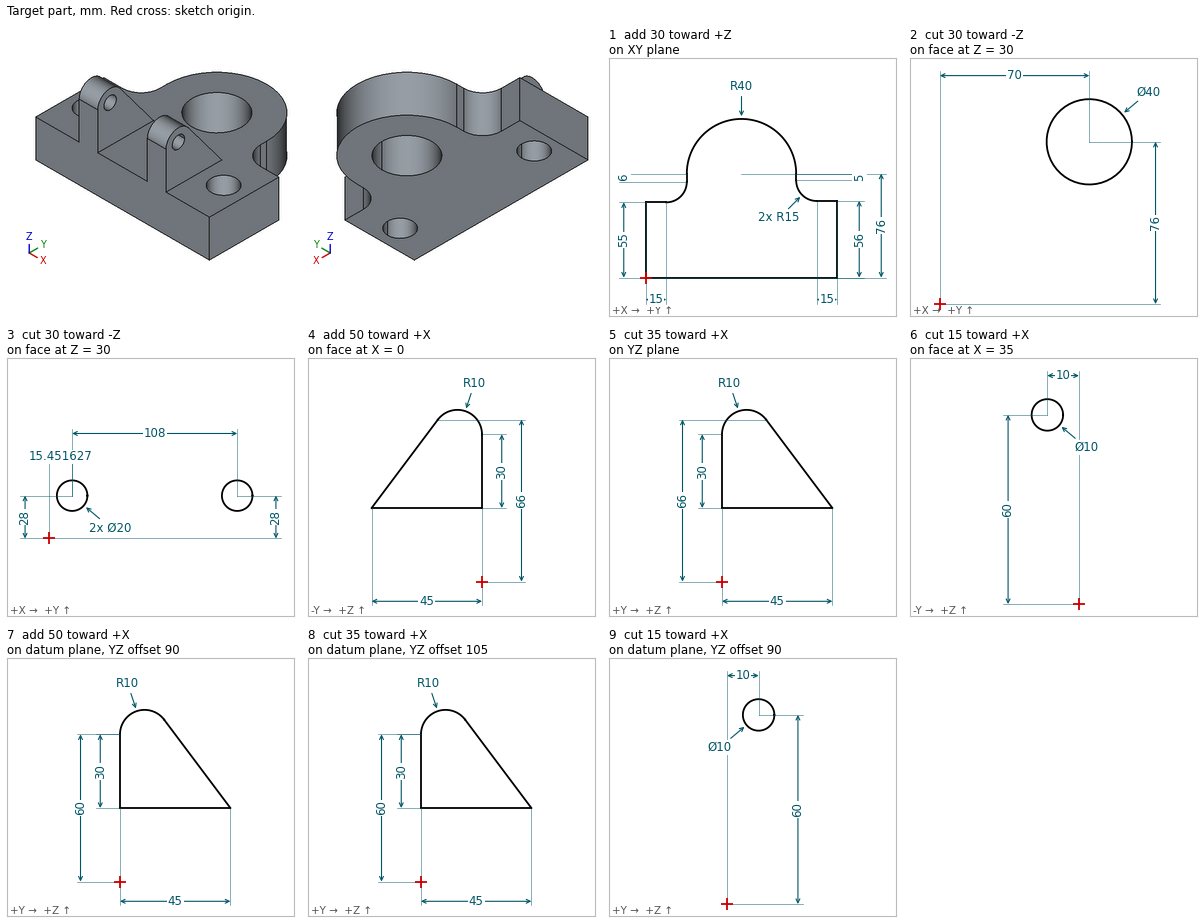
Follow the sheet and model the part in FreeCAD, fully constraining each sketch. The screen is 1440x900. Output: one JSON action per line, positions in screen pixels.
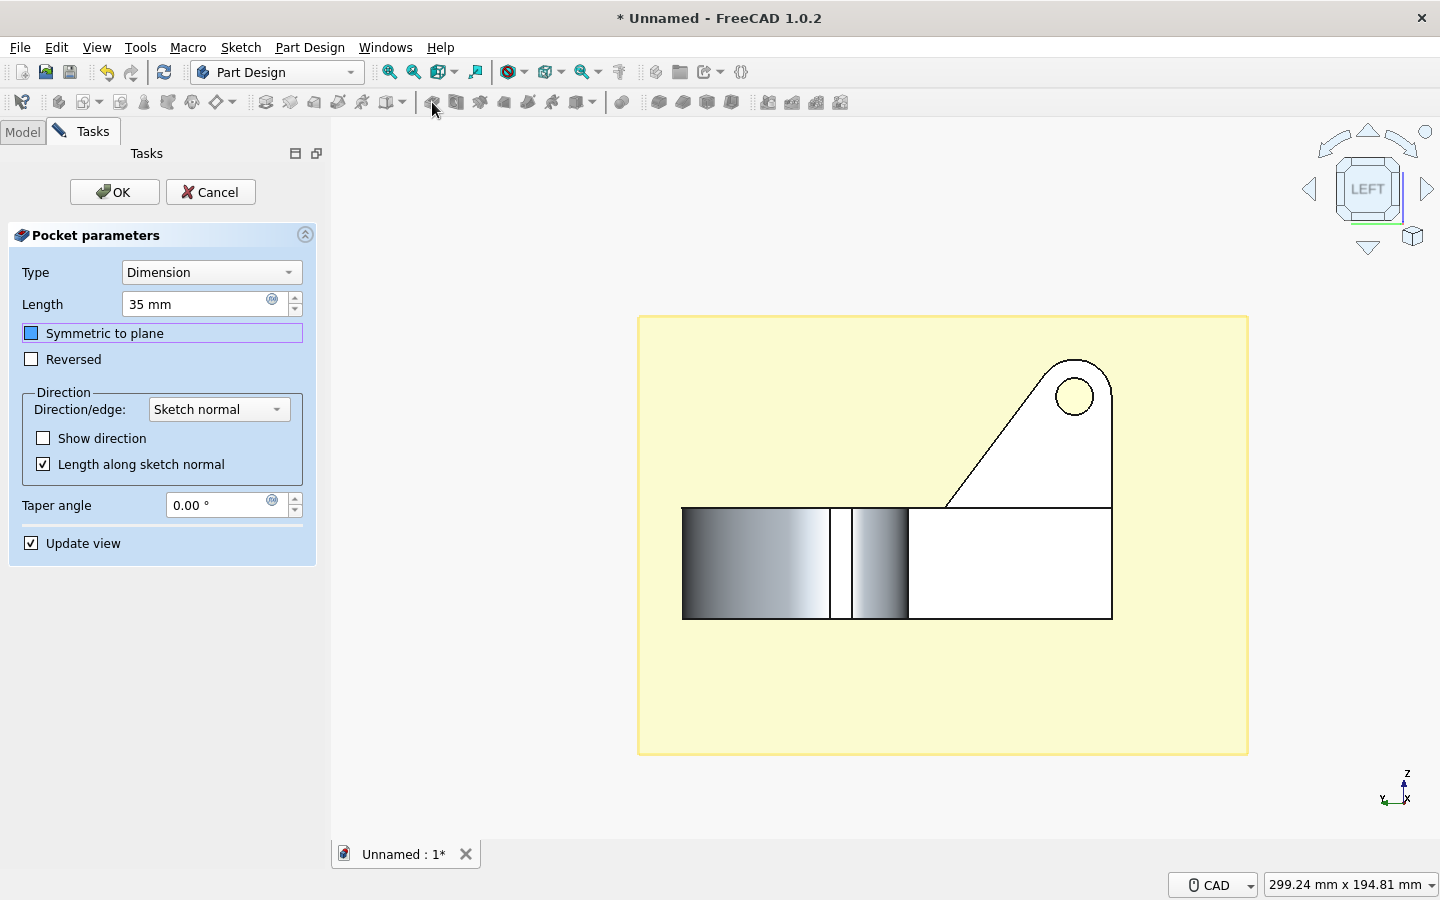
{"action": "left_click", "coordinate": [30, 359]}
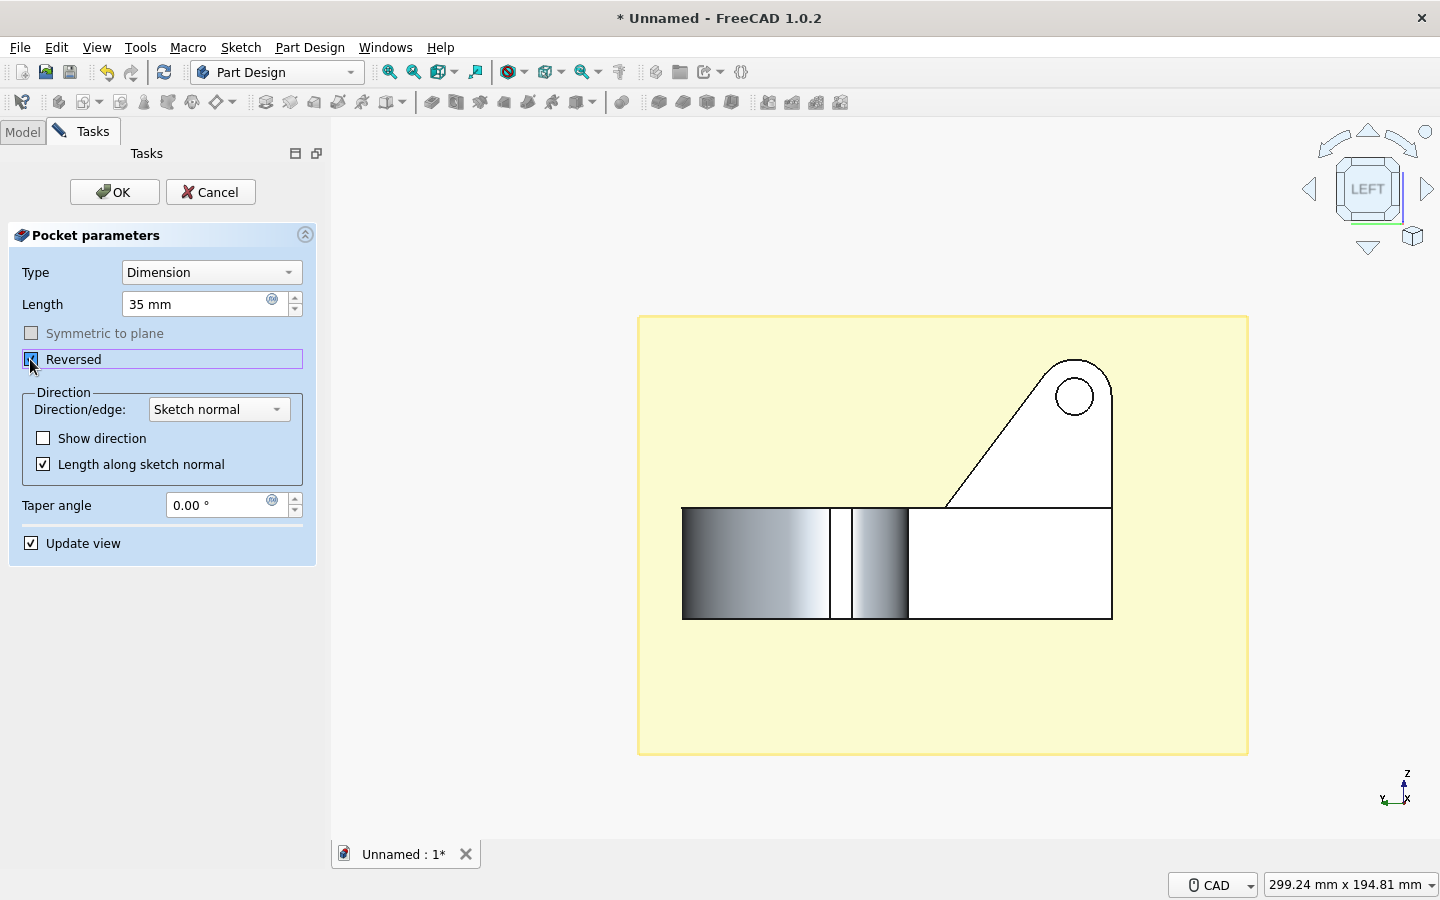
{"action": "left_click", "coordinate": [115, 192]}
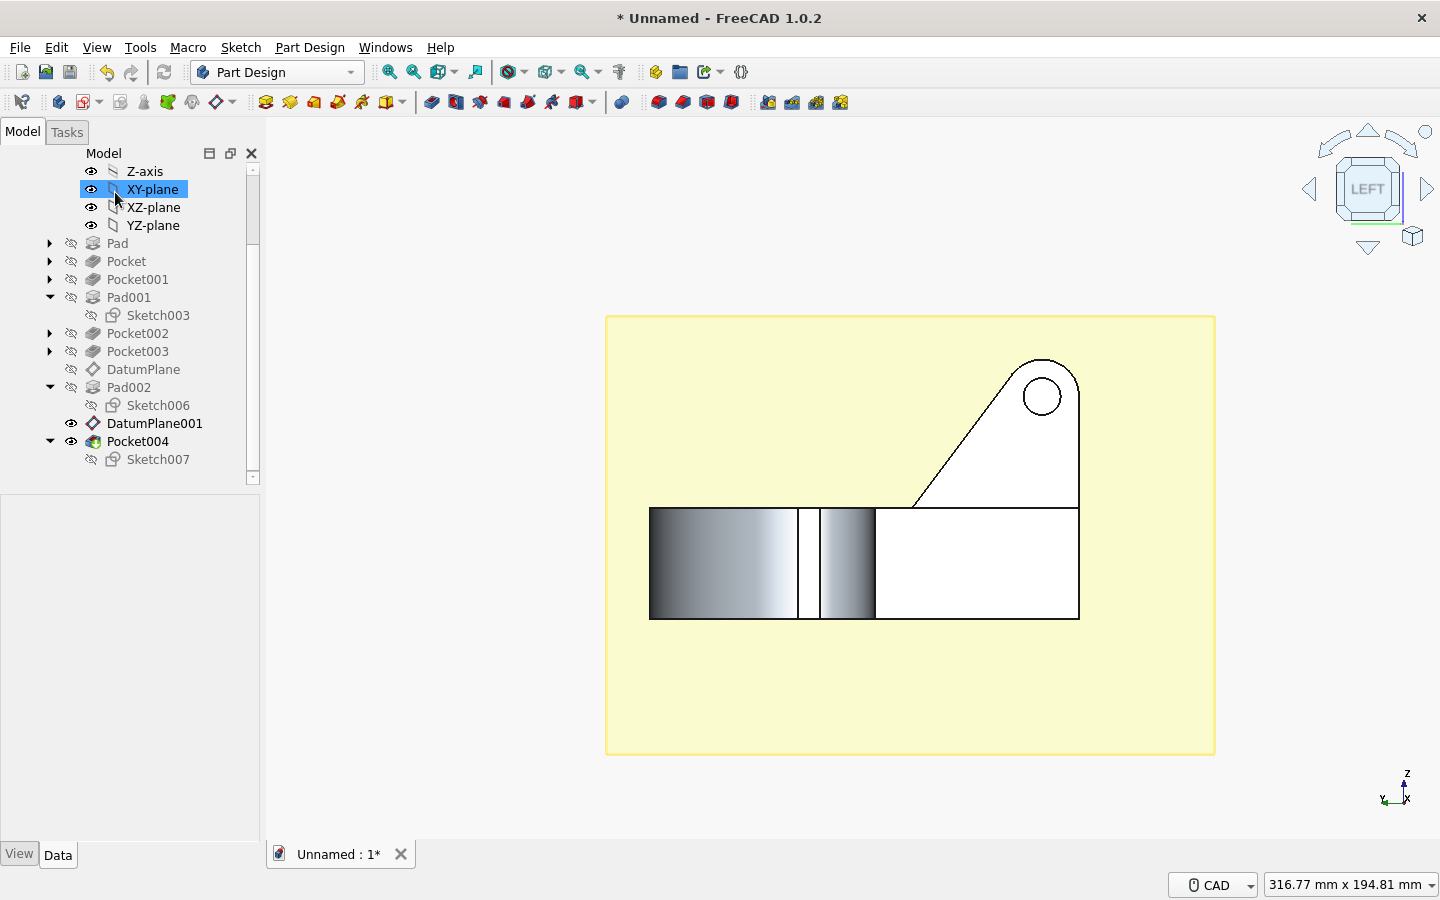
{"action": "left_click", "coordinate": [116, 423]}
{"action": "key", "text": "space"}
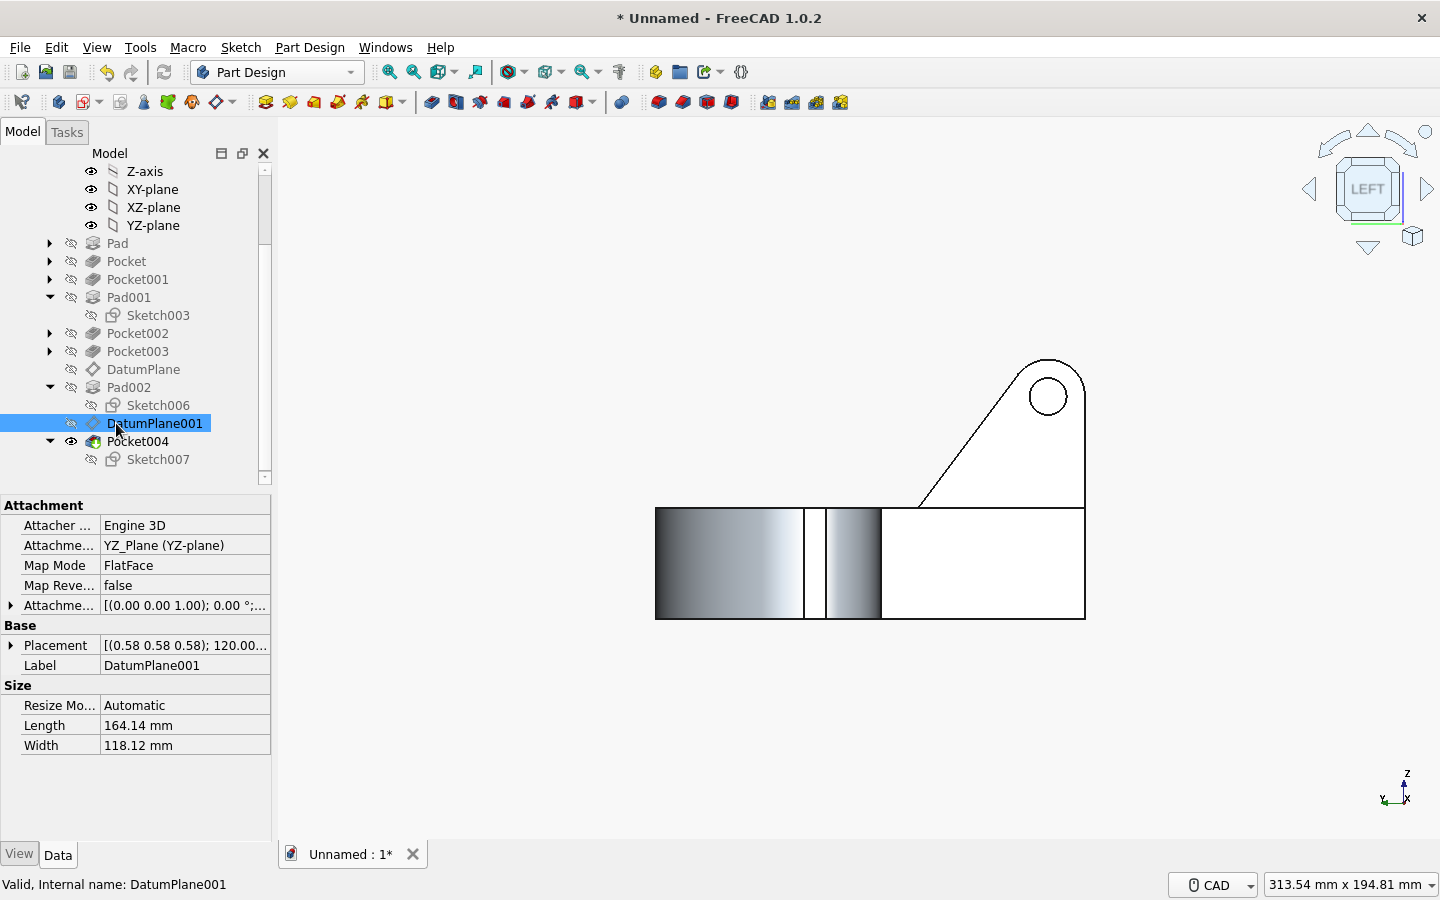
{"action": "key", "text": "v f"}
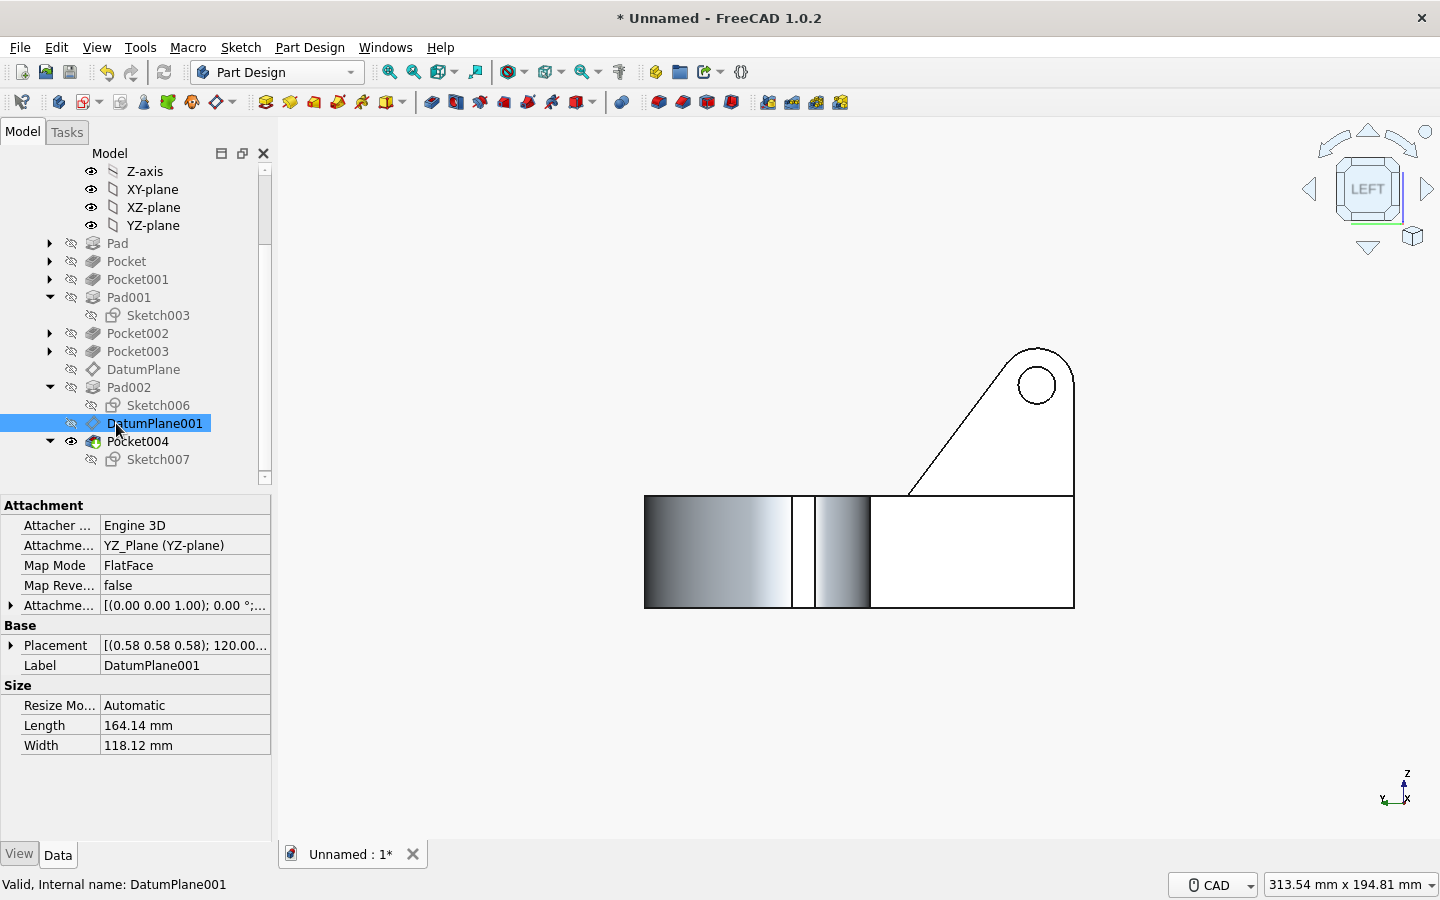
{"action": "key", "text": "2"}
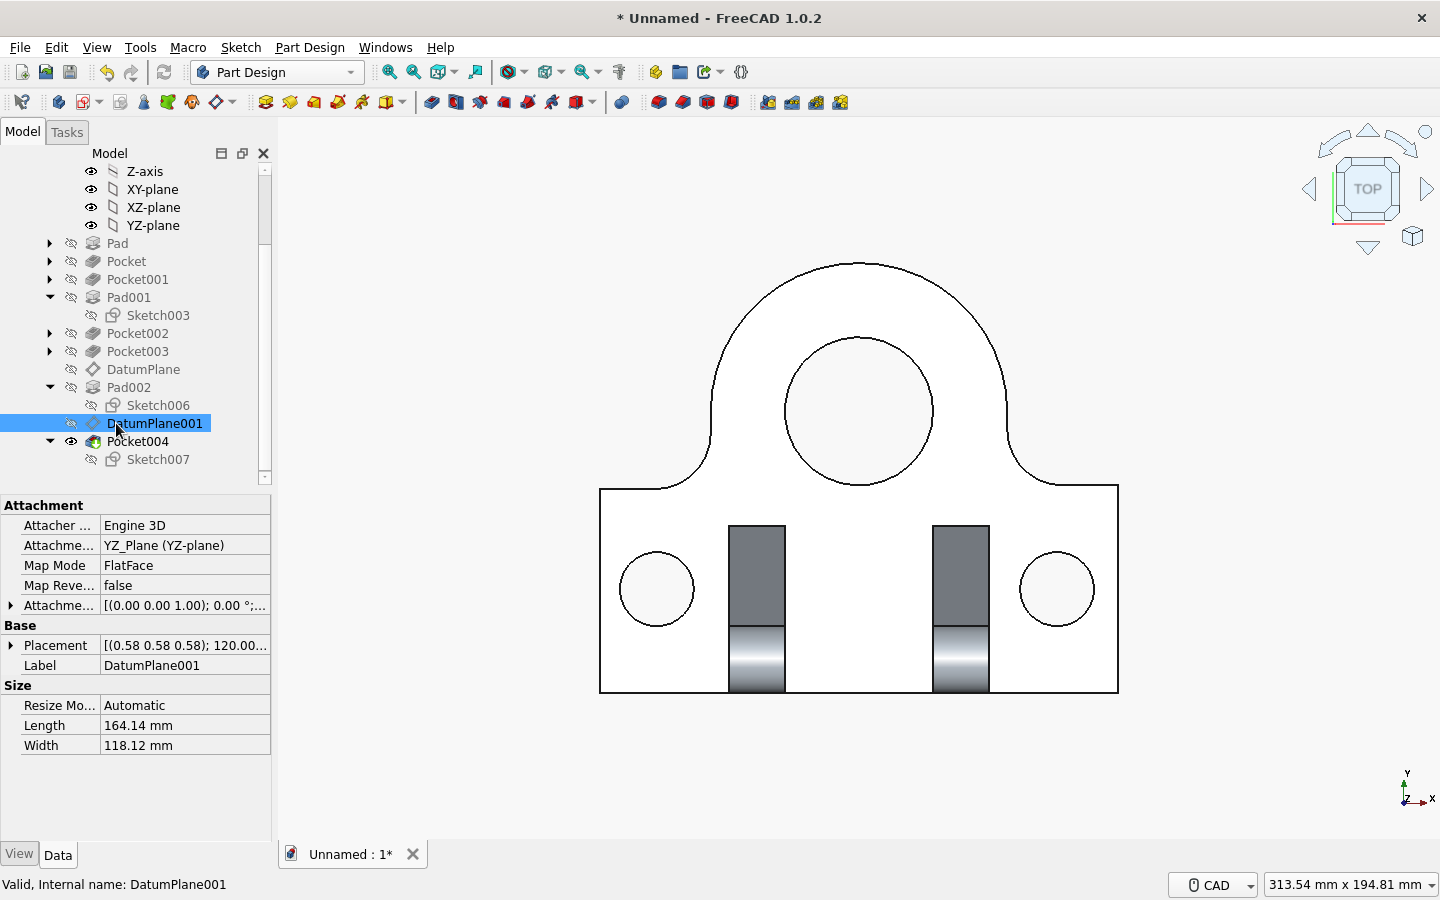
{"action": "key", "text": "6"}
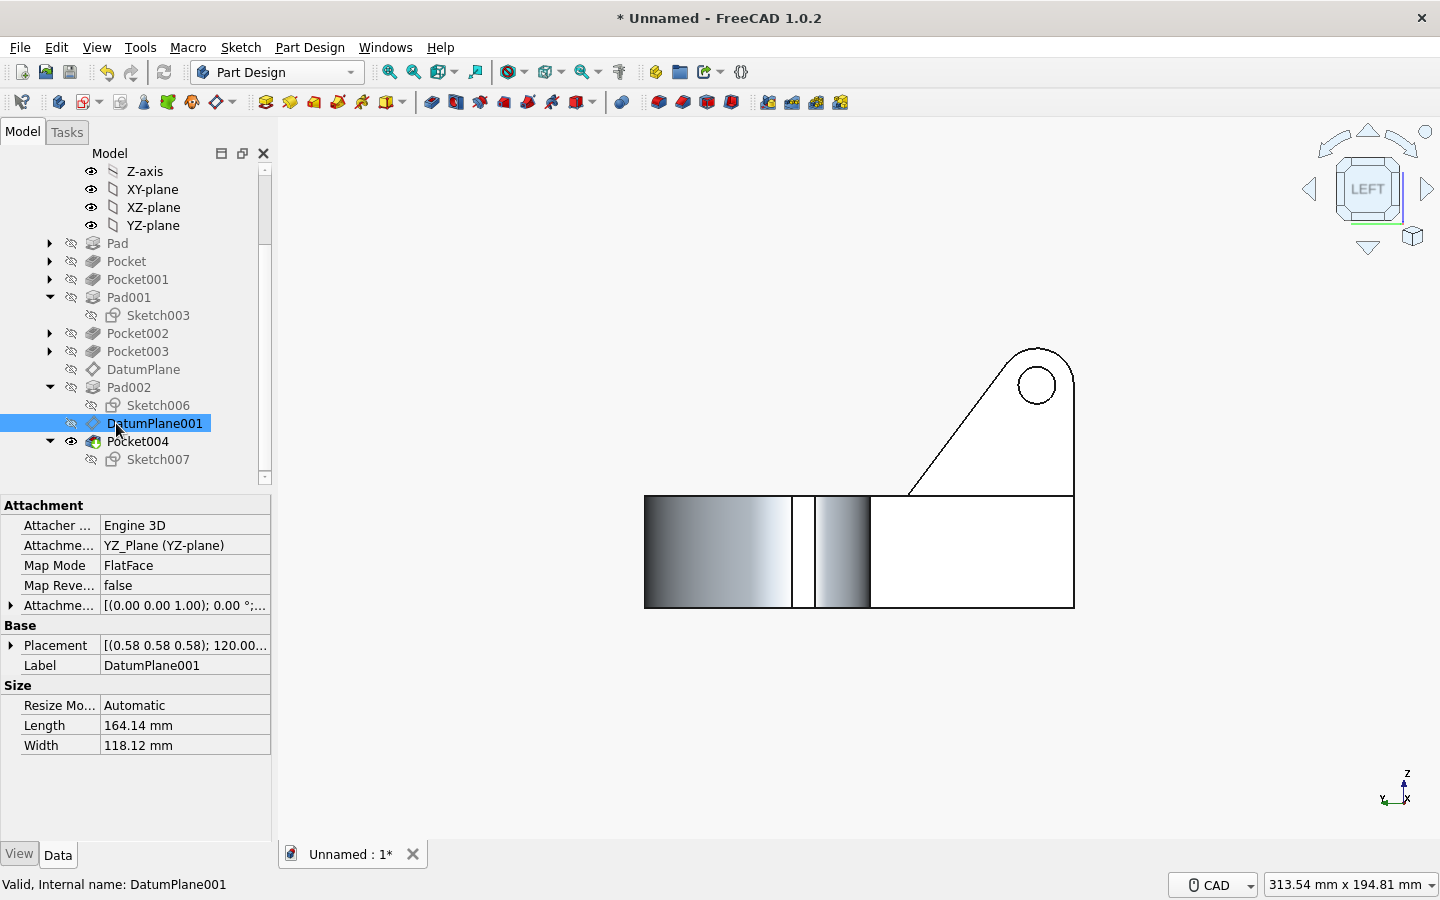
{"action": "left_click", "coordinate": [390, 72]}